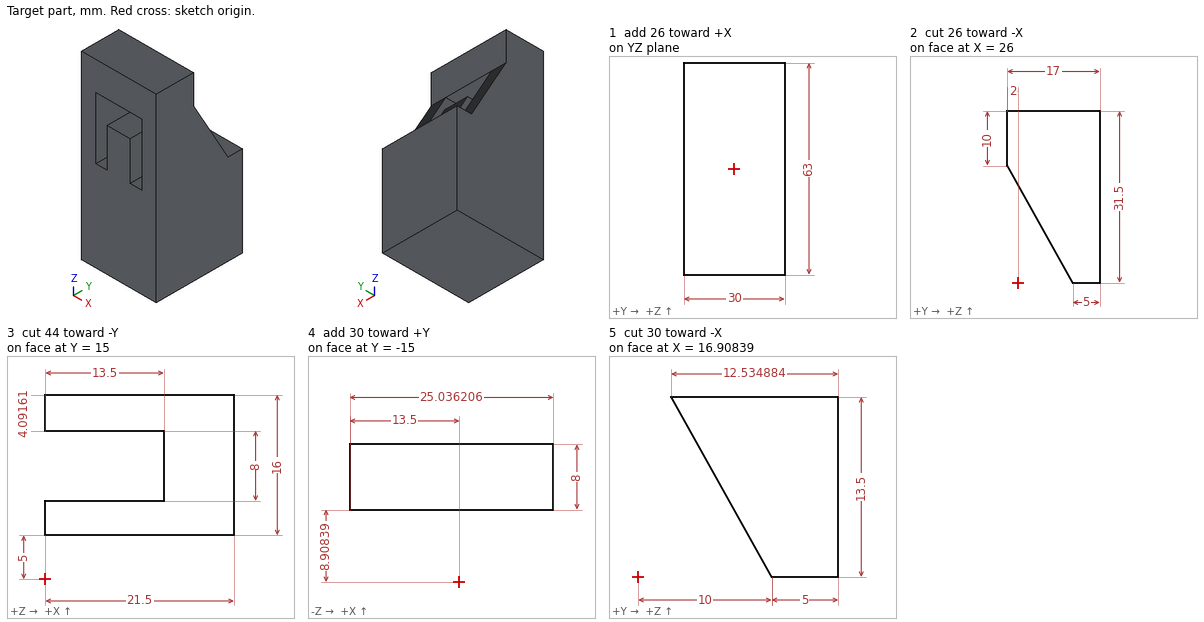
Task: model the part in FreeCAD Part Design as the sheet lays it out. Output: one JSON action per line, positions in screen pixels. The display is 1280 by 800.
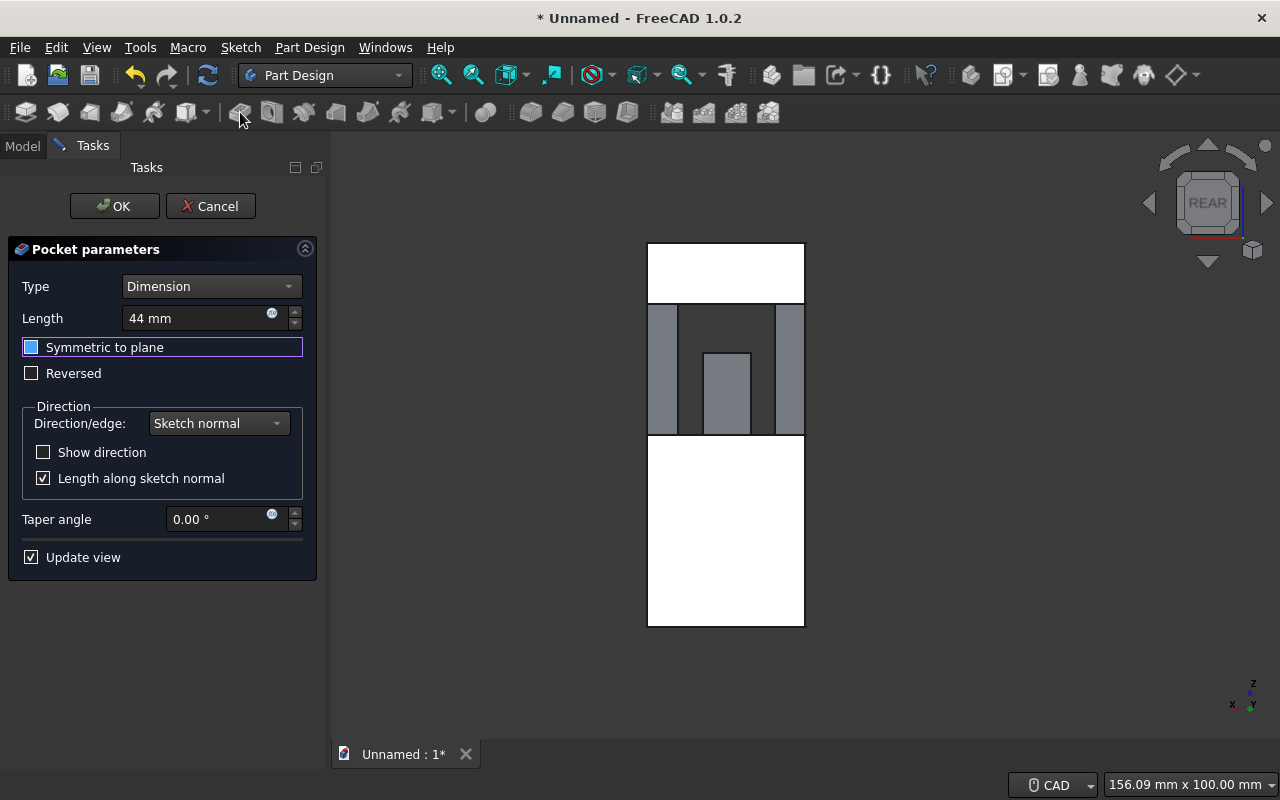
{"action": "left_click", "coordinate": [115, 206]}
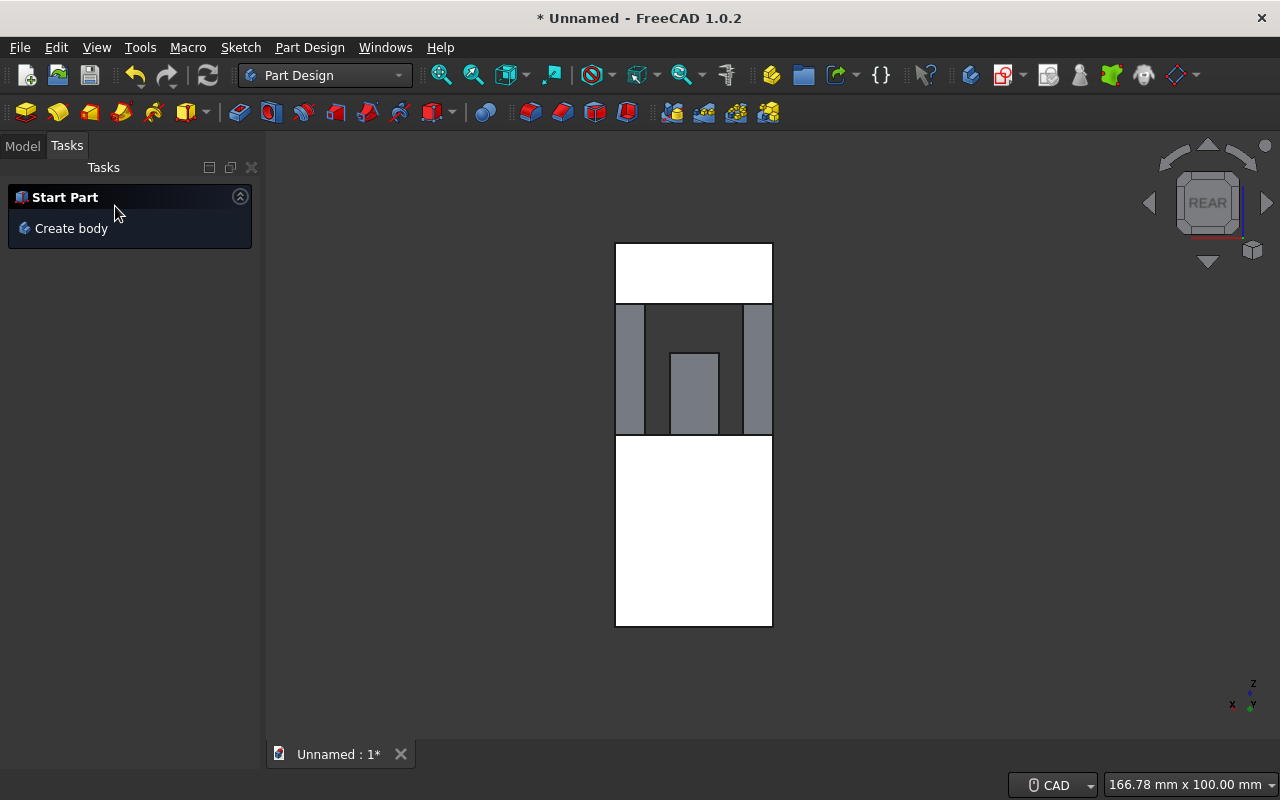
{"action": "key", "text": "0"}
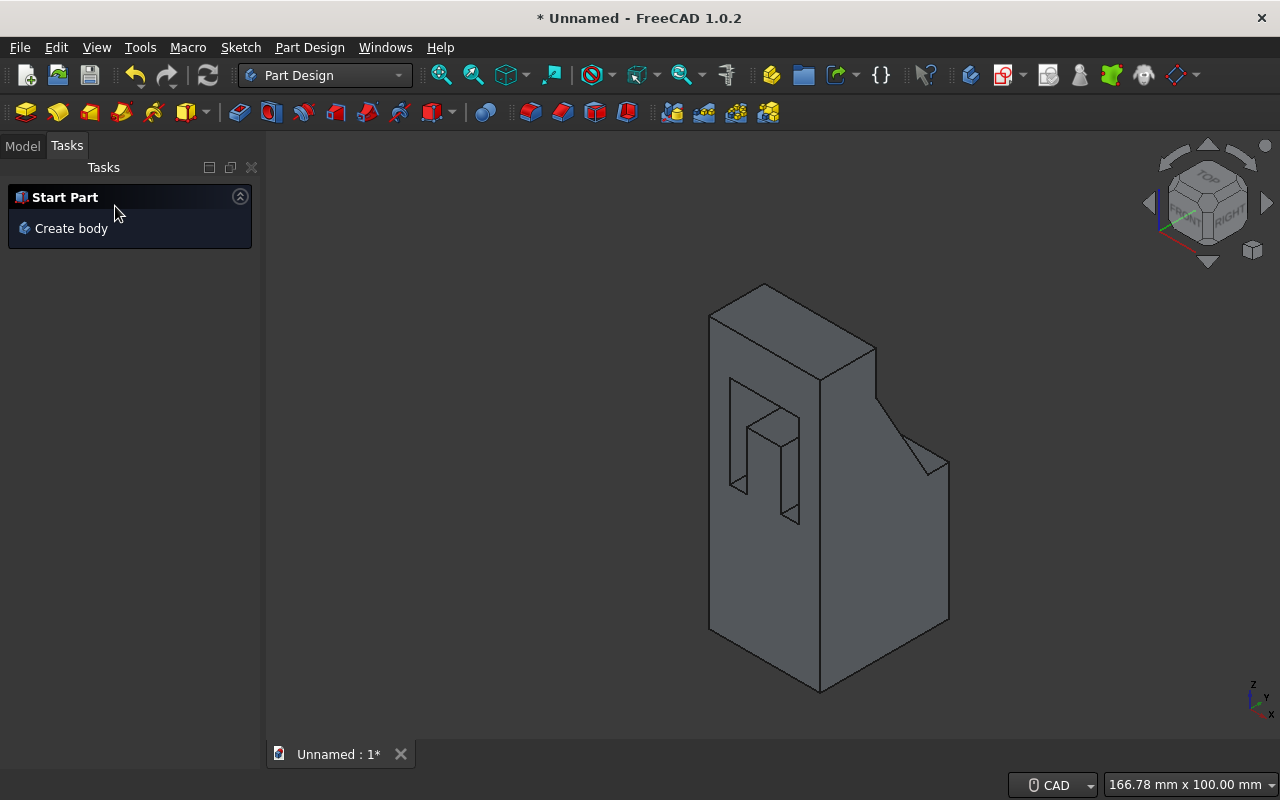
{"action": "left_click", "coordinate": [764, 593]}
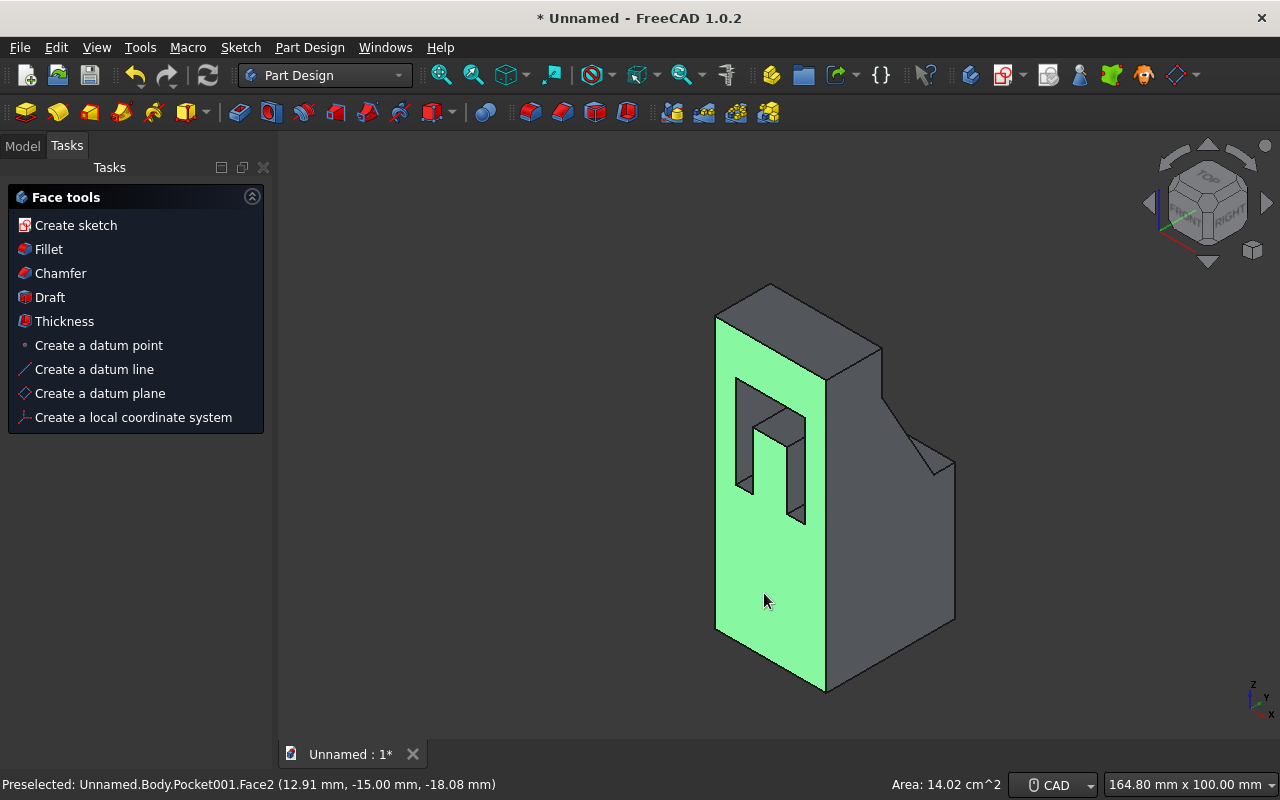
{"action": "left_click", "coordinate": [1004, 76]}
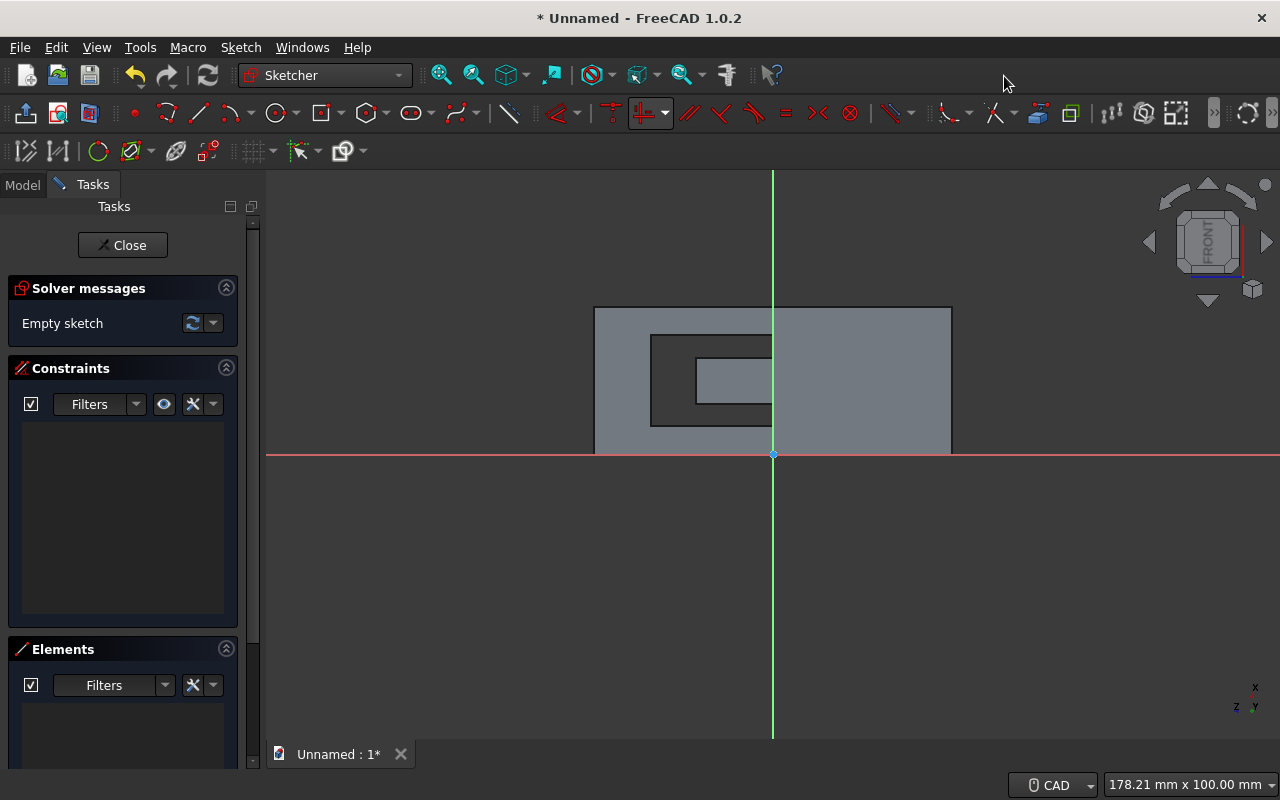
{"action": "scroll", "coordinate": [788, 391], "scroll_direction": "up", "scroll_amount": 7}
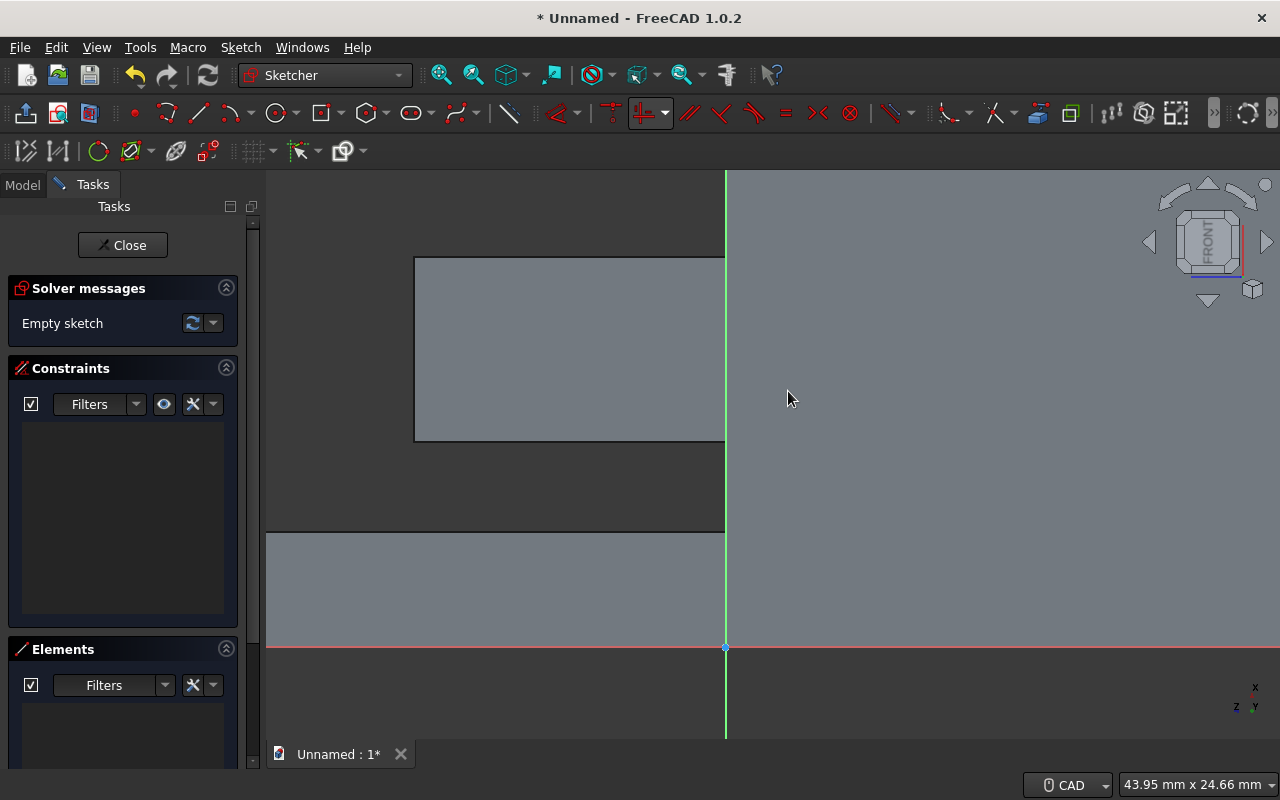
{"action": "key", "text": "g r"}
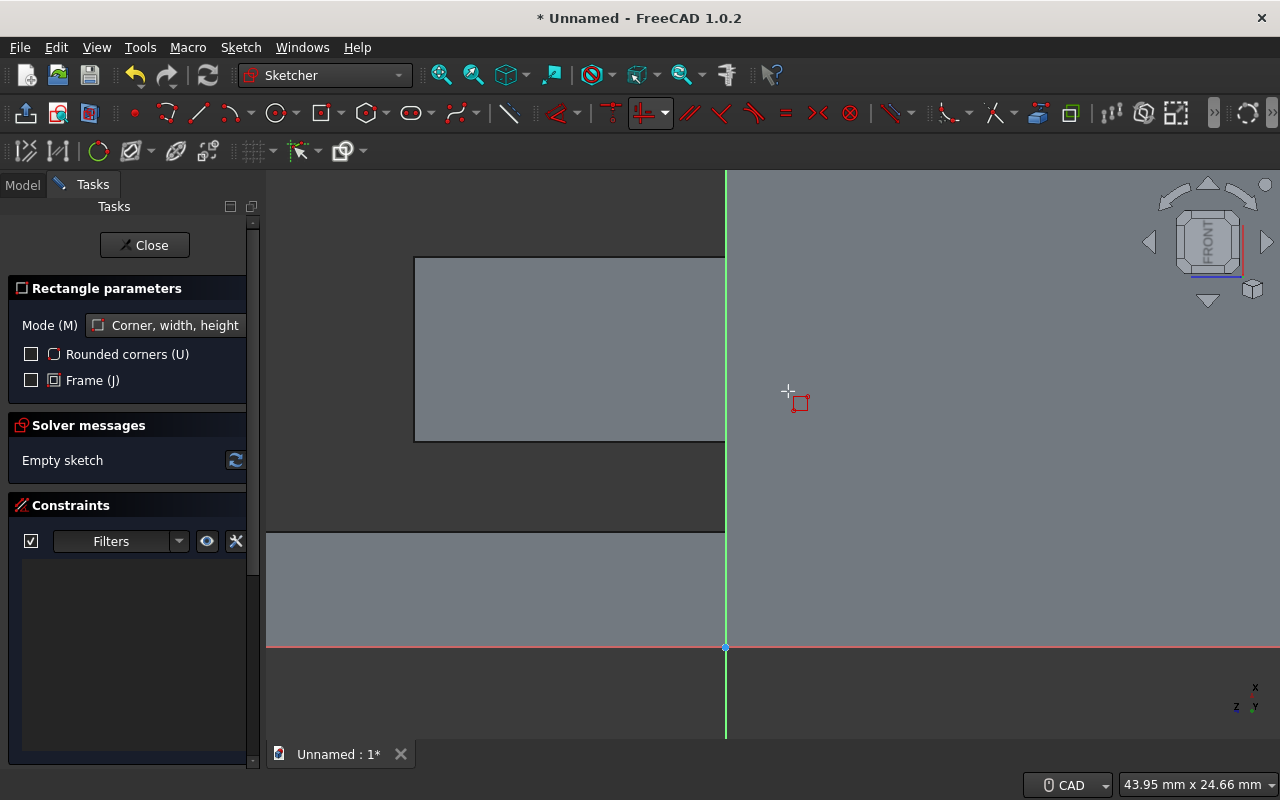
{"action": "left_click", "coordinate": [414, 257]}
{"action": "mouse_move", "coordinate": [992, 442]}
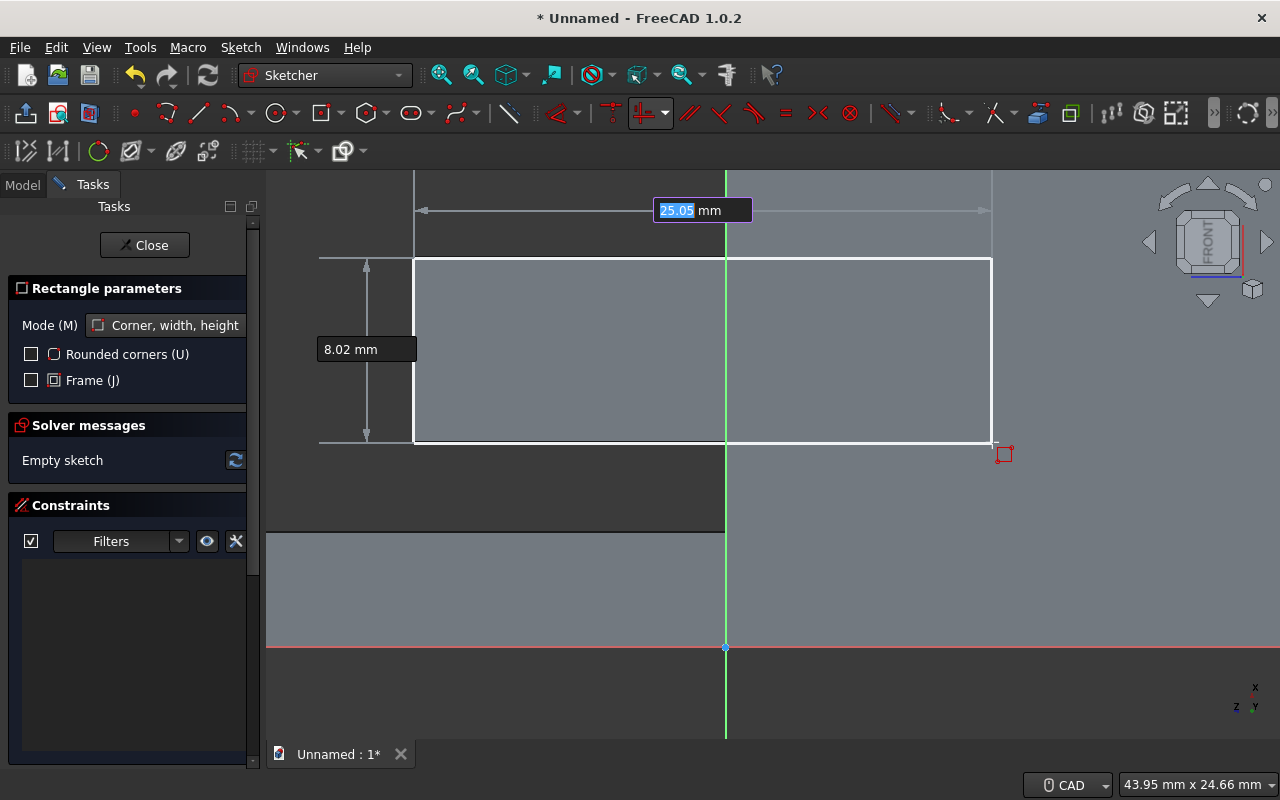
{"action": "type", "text": "25.036206"}
{"action": "key", "text": "Tab"}
{"action": "type", "text": "8"}
{"action": "key", "text": "Return"}
{"action": "key", "text": "Escape"}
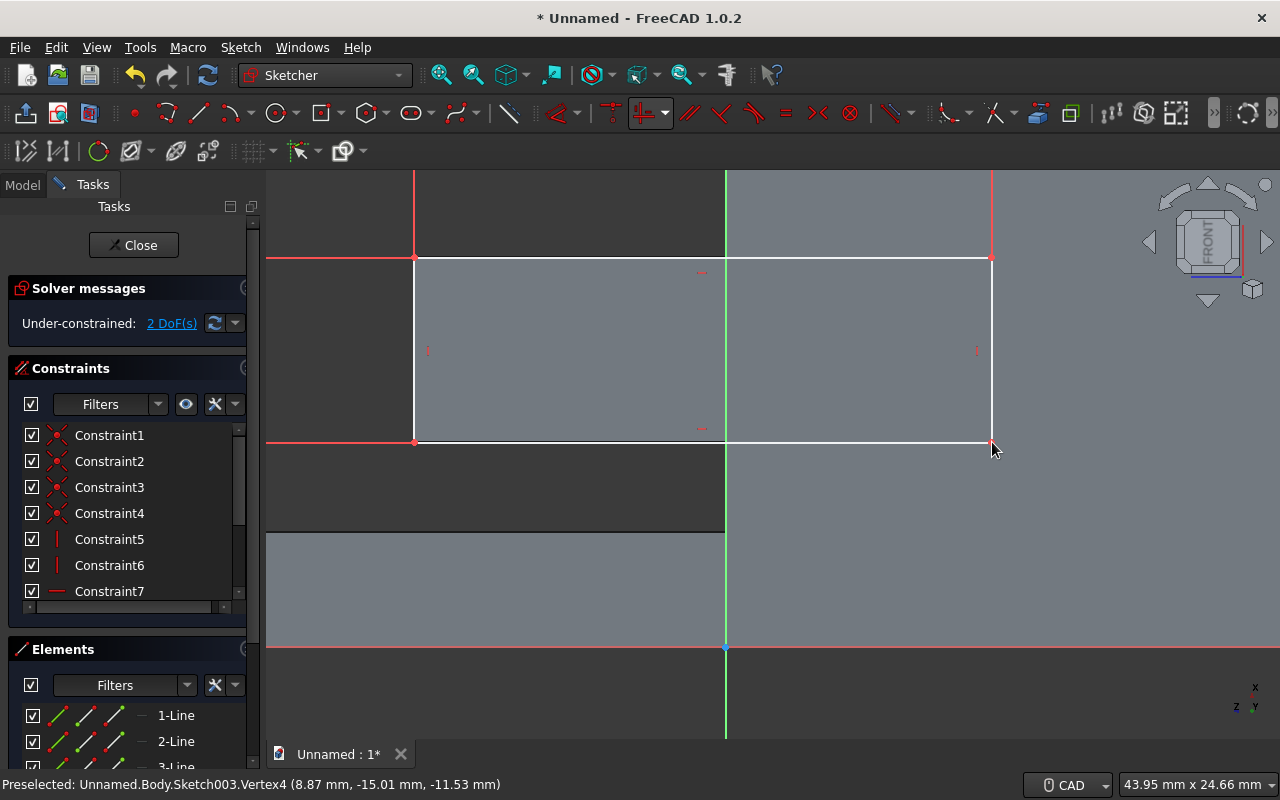
{"action": "left_click", "coordinate": [556, 114]}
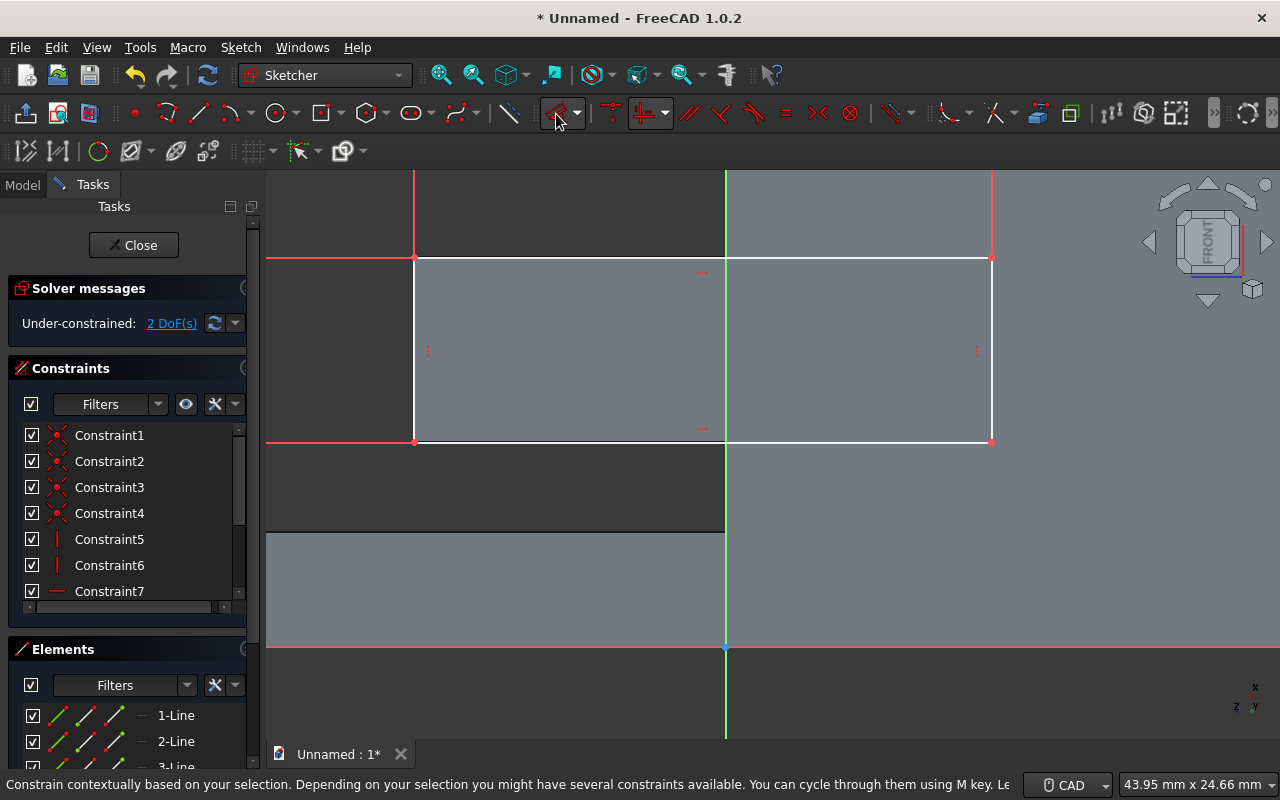
{"action": "left_click", "coordinate": [414, 258]}
{"action": "left_click", "coordinate": [570, 681]}